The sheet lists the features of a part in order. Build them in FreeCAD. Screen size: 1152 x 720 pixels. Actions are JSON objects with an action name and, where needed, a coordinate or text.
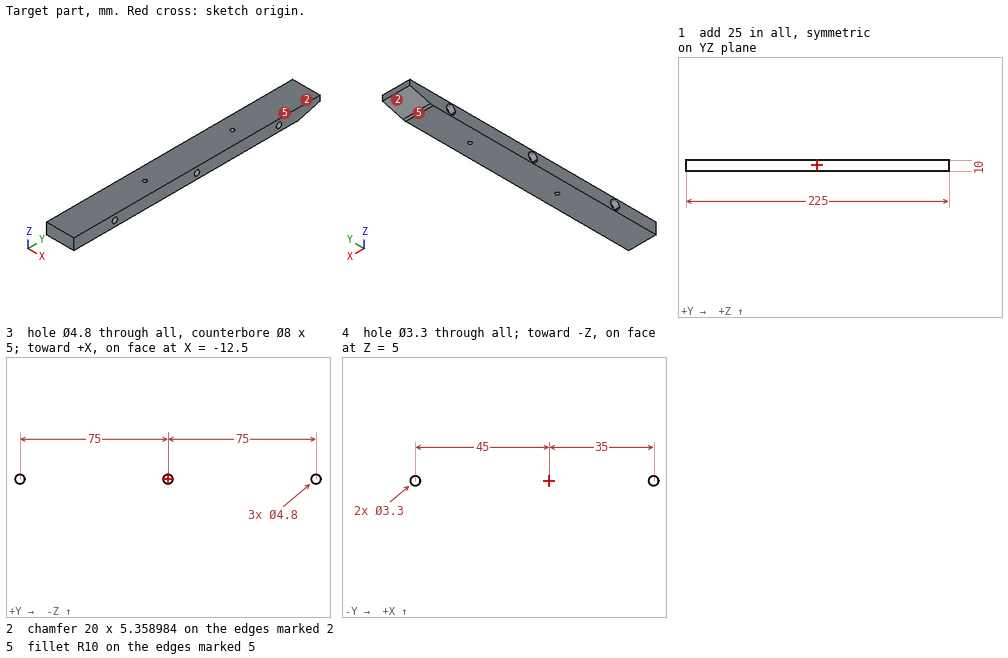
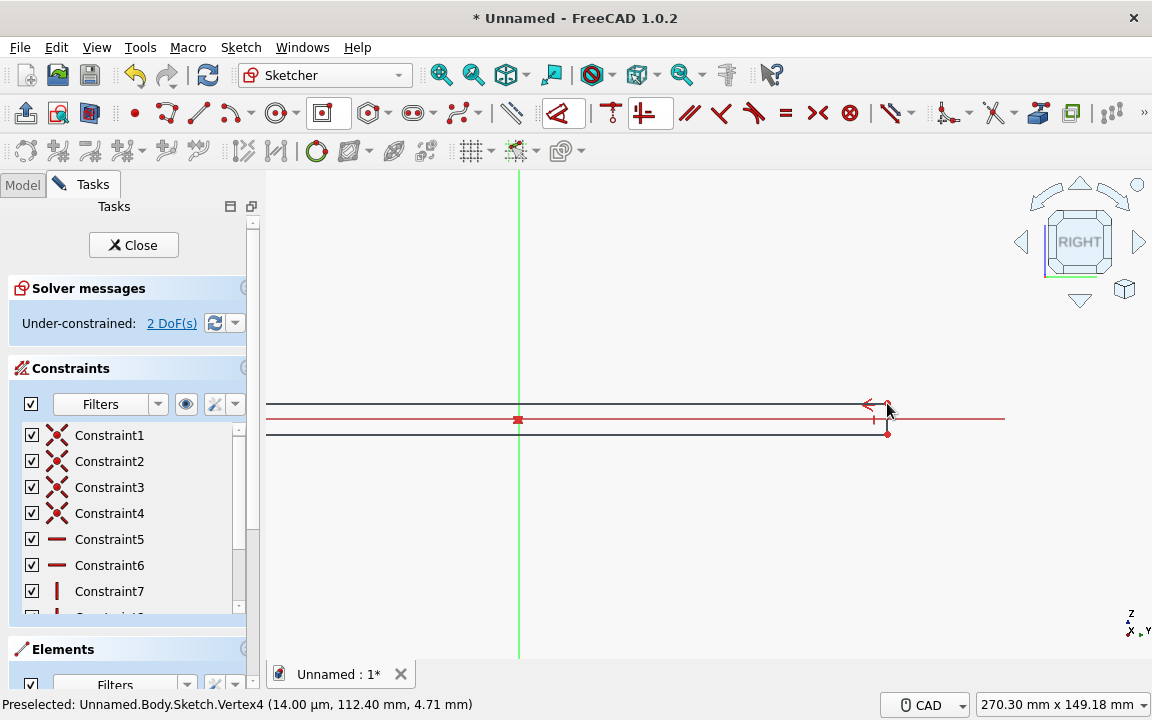
{"action": "left_click", "coordinate": [558, 114]}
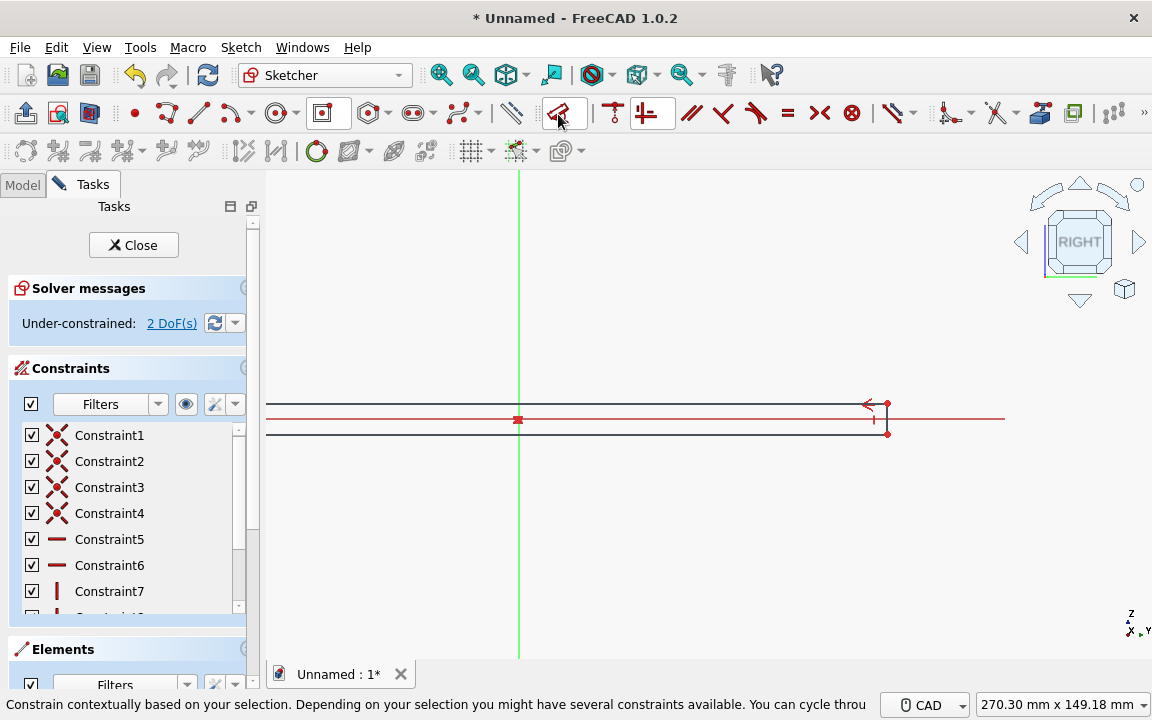
{"action": "left_click", "coordinate": [887, 423]}
{"action": "left_click", "coordinate": [921, 412]}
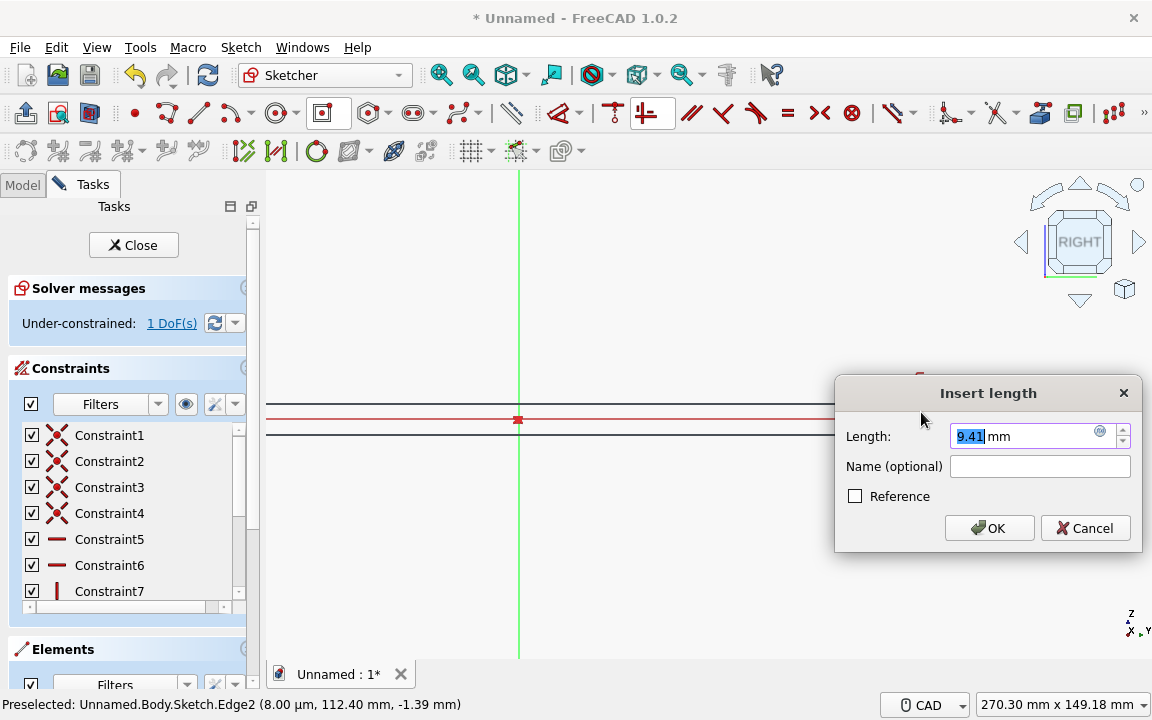
{"action": "type", "text": "10"}
{"action": "key", "text": "Return"}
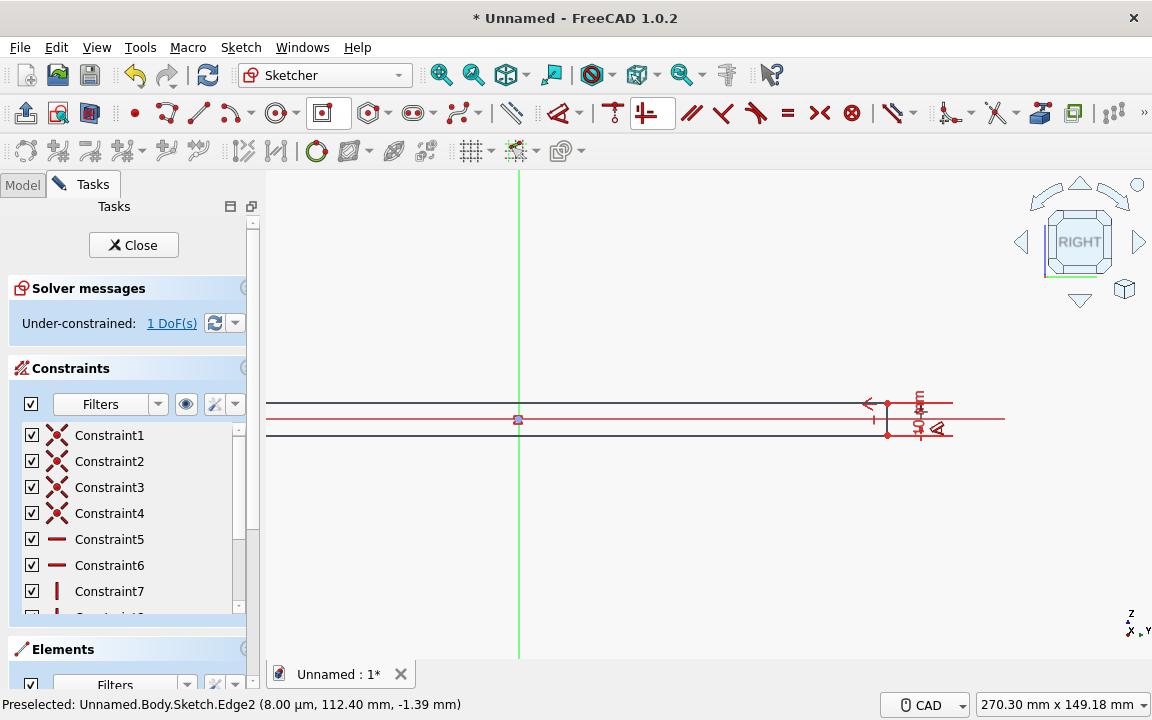
{"action": "left_click", "coordinate": [371, 436]}
{"action": "left_click", "coordinate": [591, 470]}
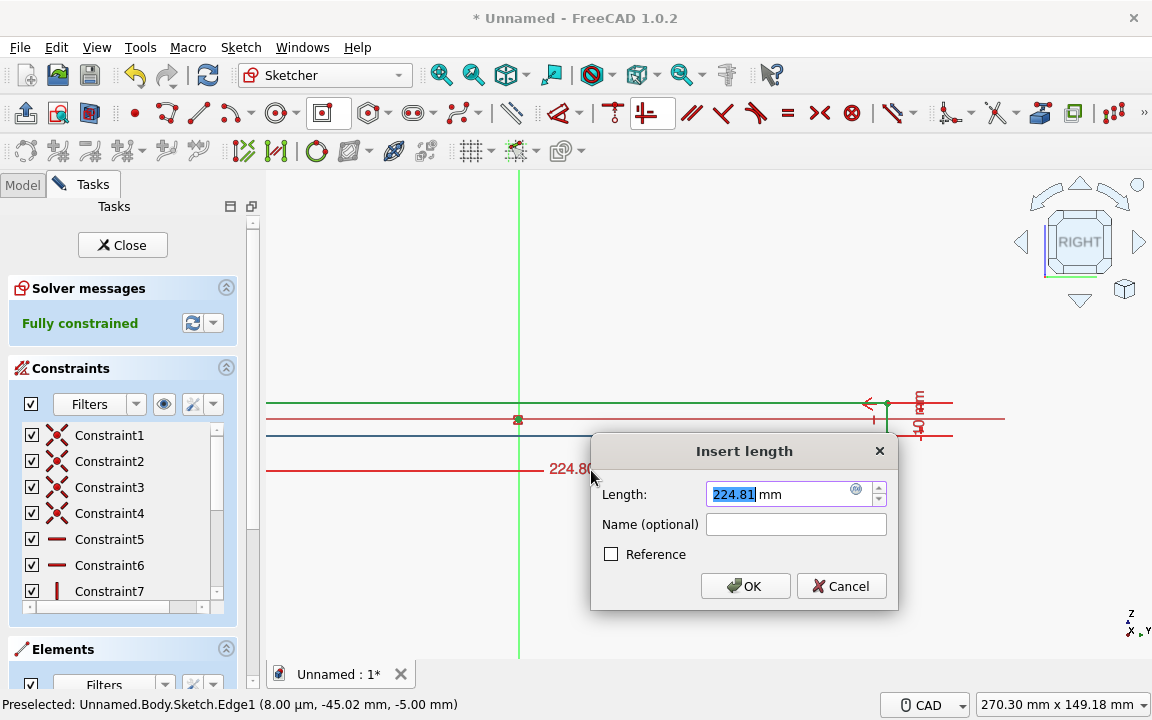
{"action": "type", "text": "225"}
{"action": "key", "text": "Return"}
{"action": "key", "text": "Escape"}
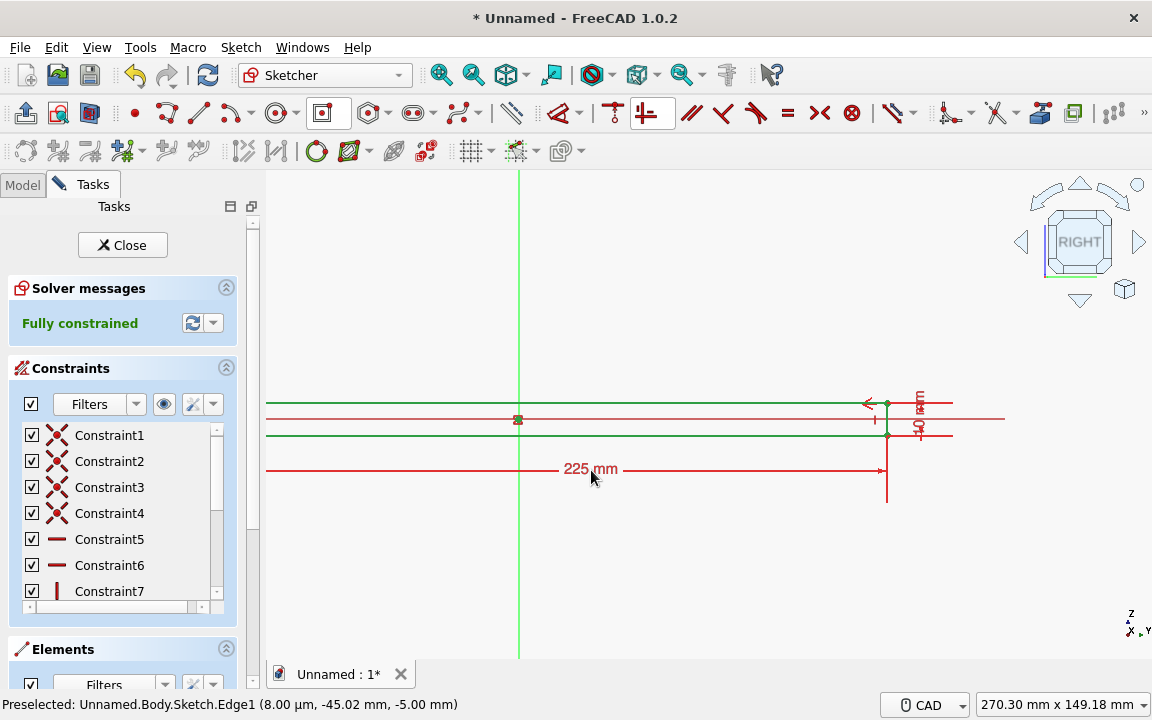
{"action": "left_click", "coordinate": [123, 245]}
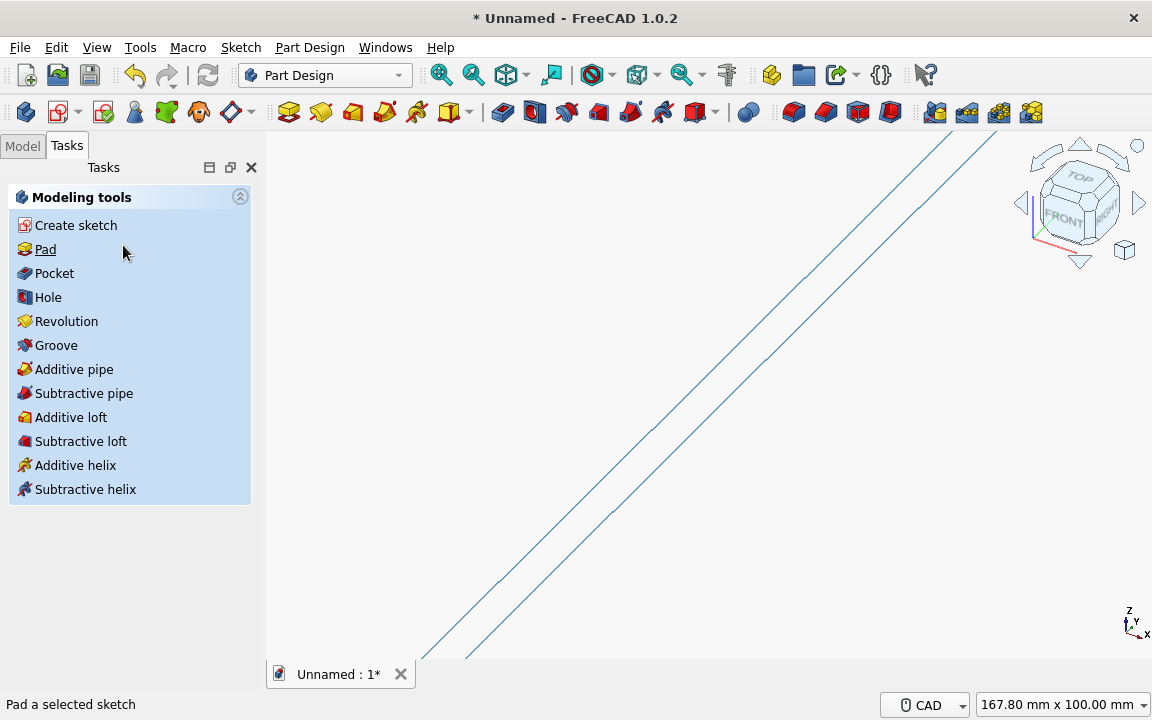
{"action": "left_click", "coordinate": [290, 112]}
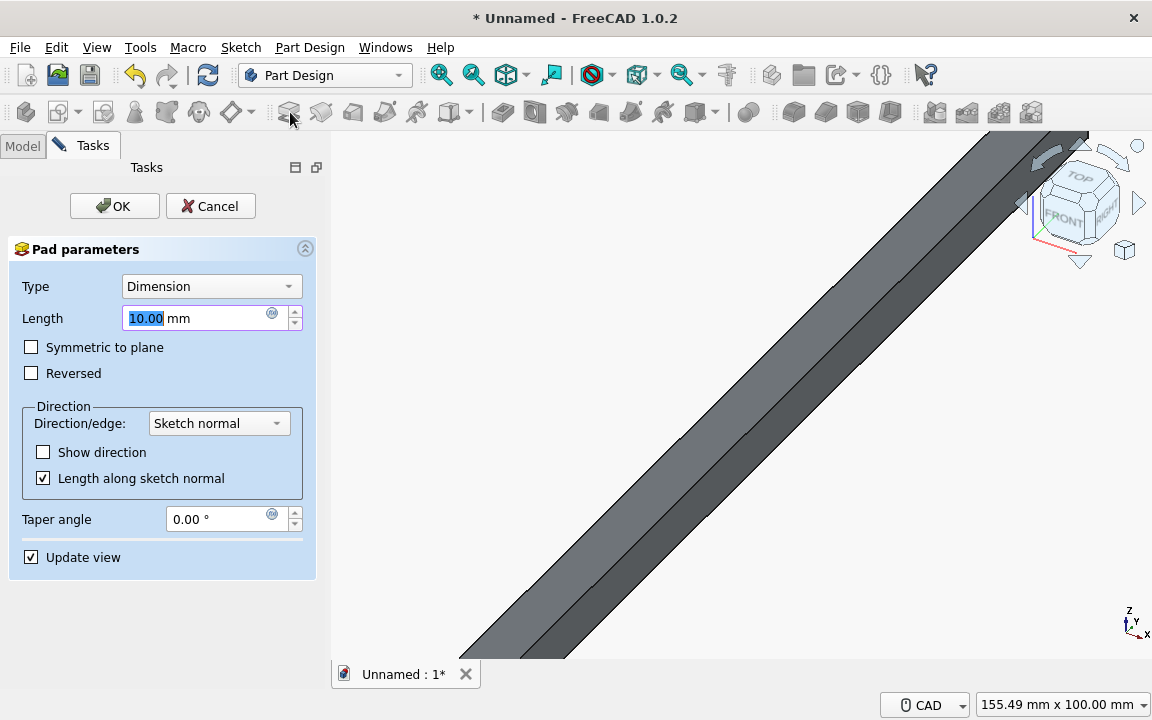
{"action": "type", "text": "25"}
{"action": "key", "text": "Tab"}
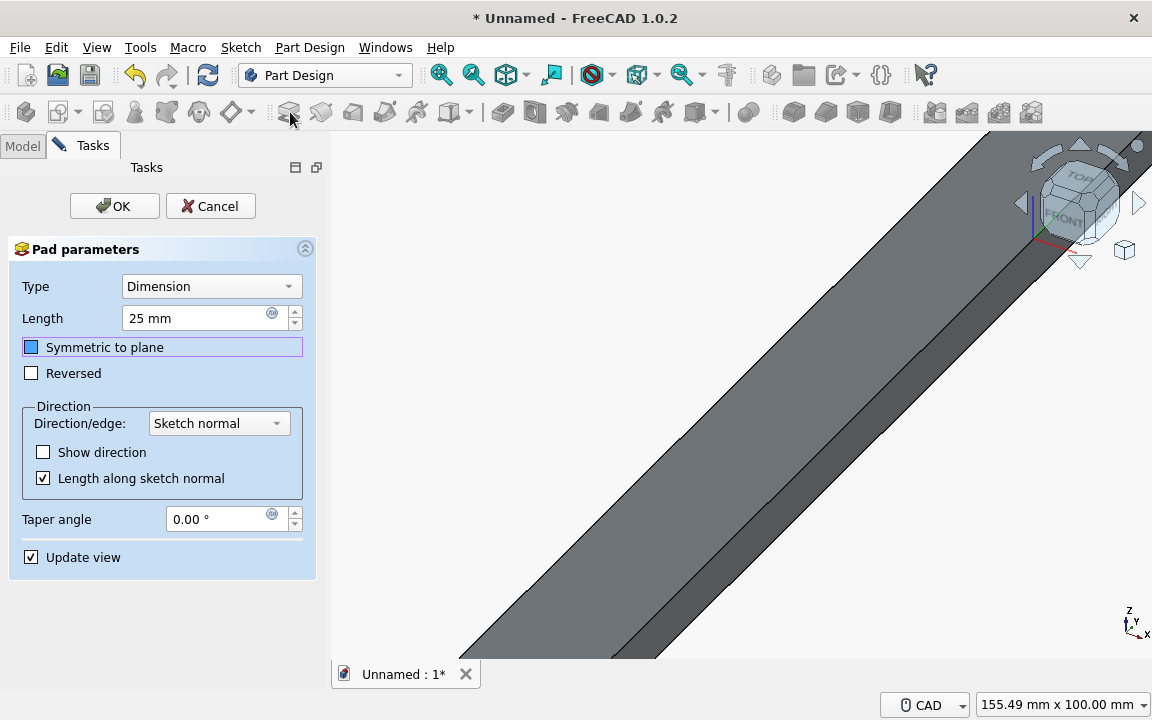
{"action": "left_click", "coordinate": [30, 347]}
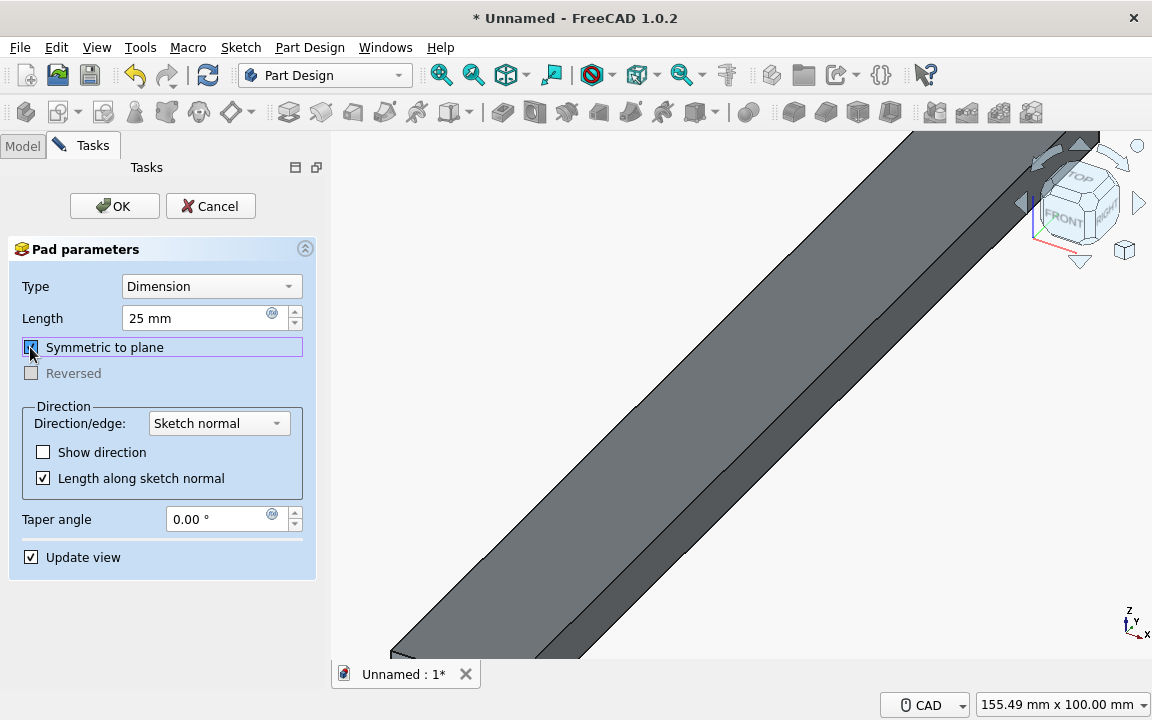
{"action": "left_click", "coordinate": [115, 206]}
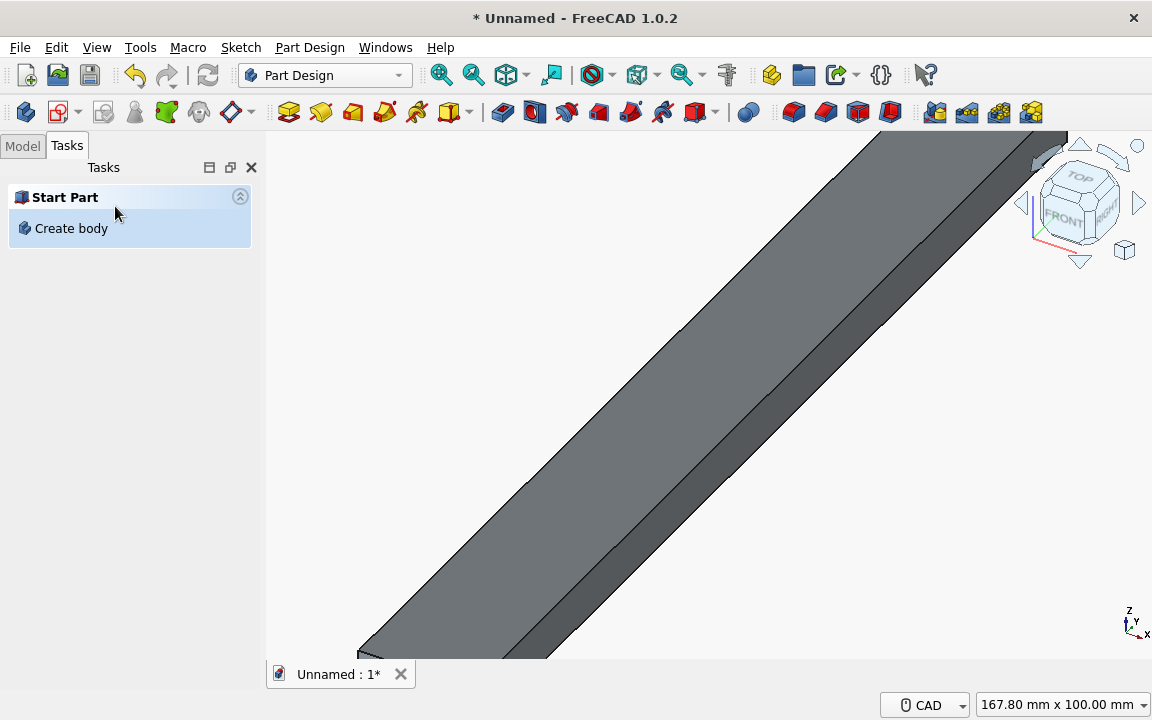
{"action": "left_click", "coordinate": [442, 76]}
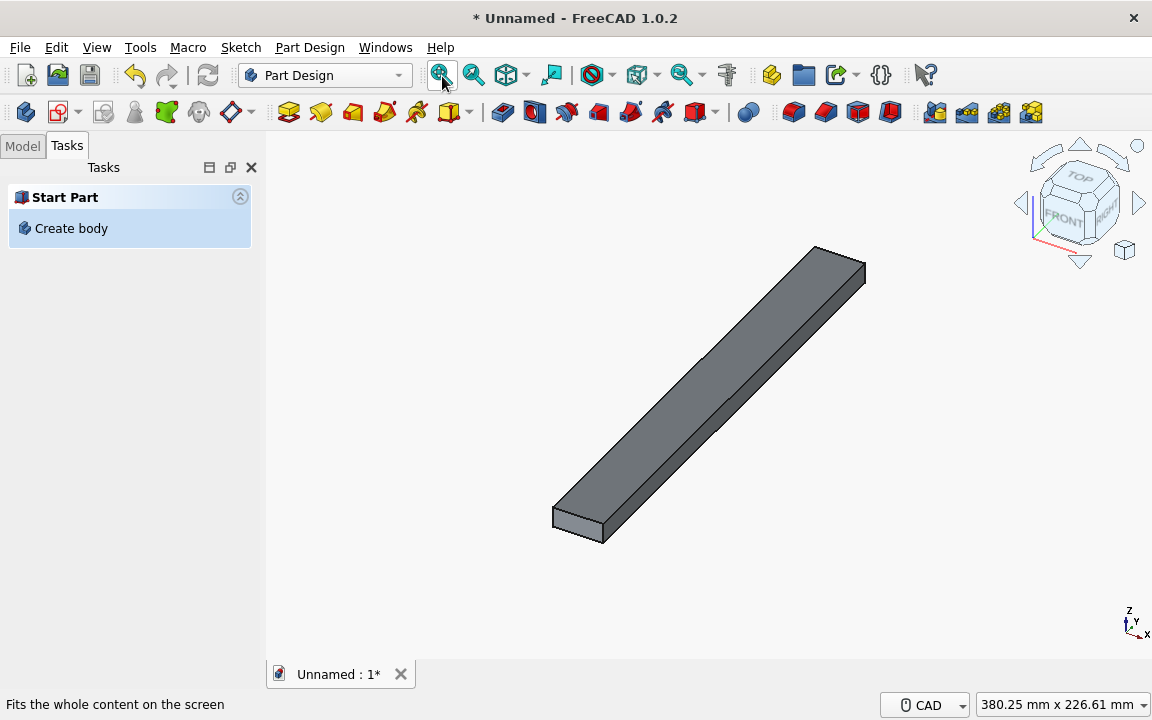
{"action": "key", "text": "0"}